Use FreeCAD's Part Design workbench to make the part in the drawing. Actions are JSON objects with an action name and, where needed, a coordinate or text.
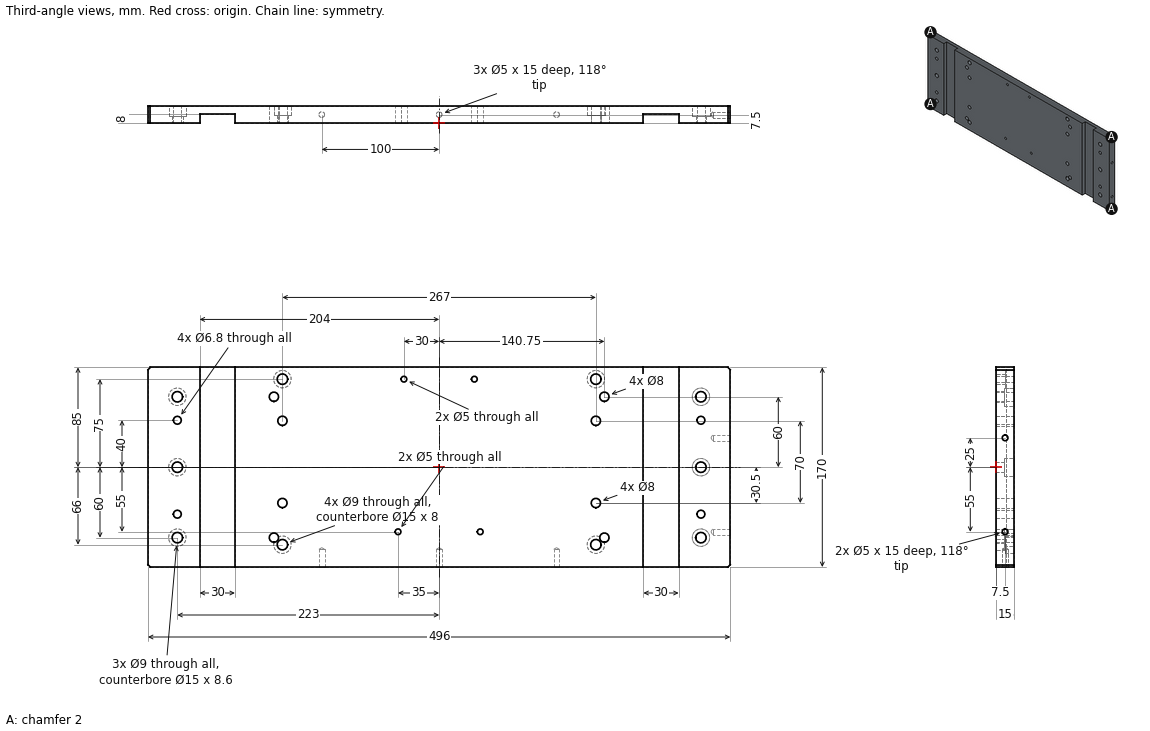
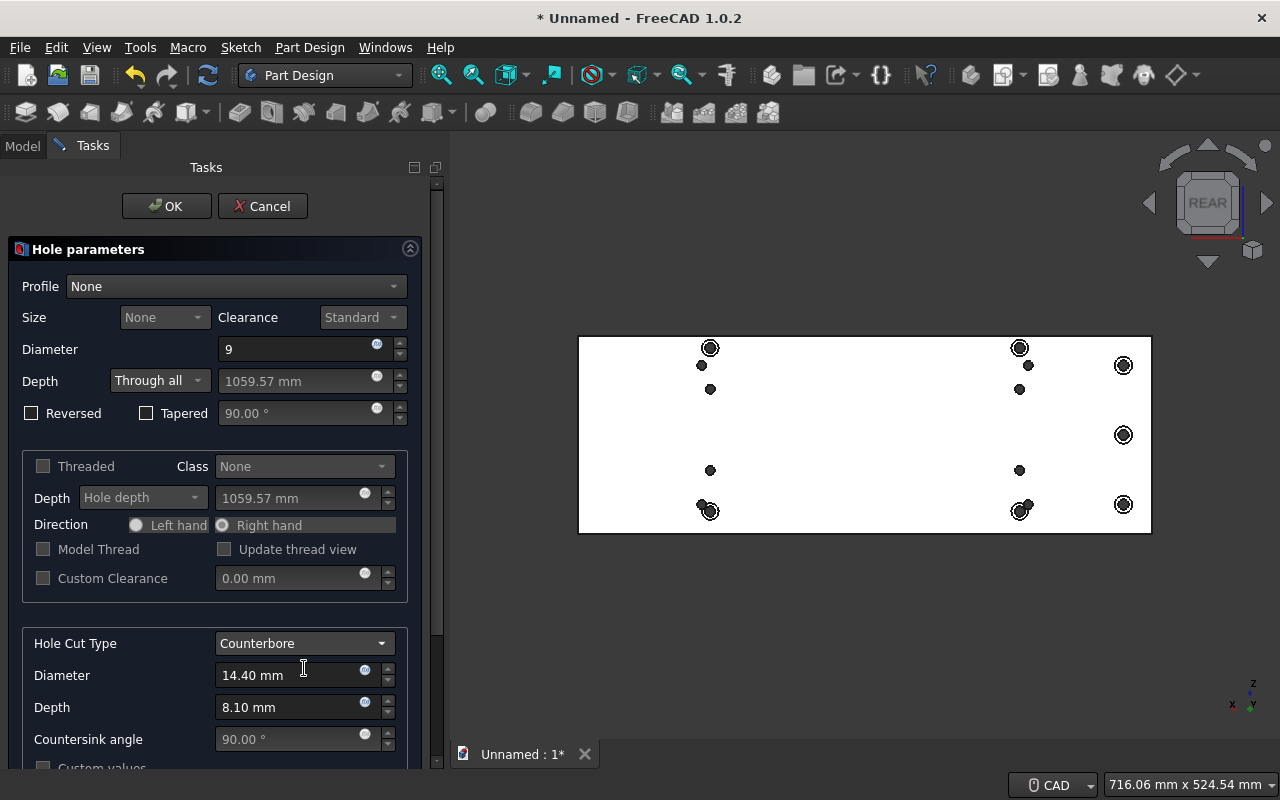
{"action": "triple_click", "coordinate": [298, 675]}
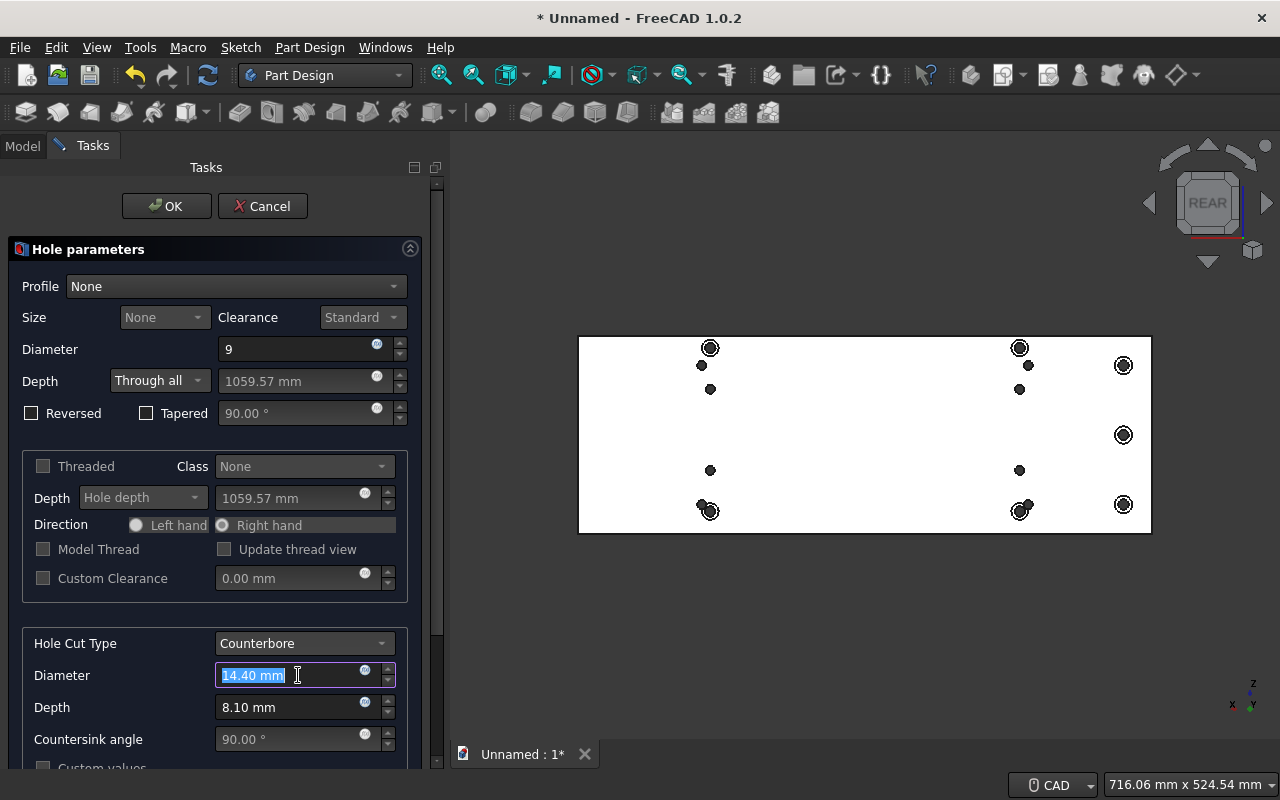
{"action": "type", "text": "15"}
{"action": "key", "text": "Tab"}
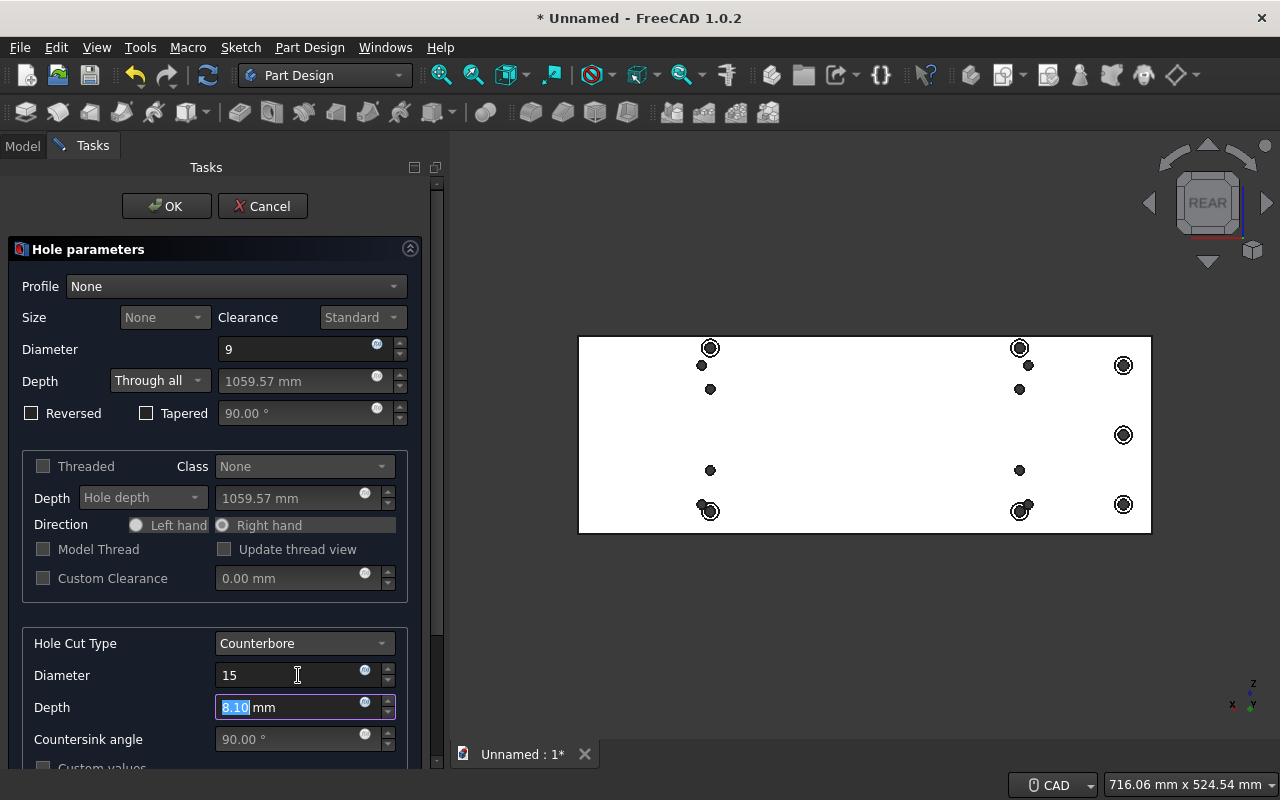
{"action": "type", "text": "8"}
{"action": "key", "text": "Tab"}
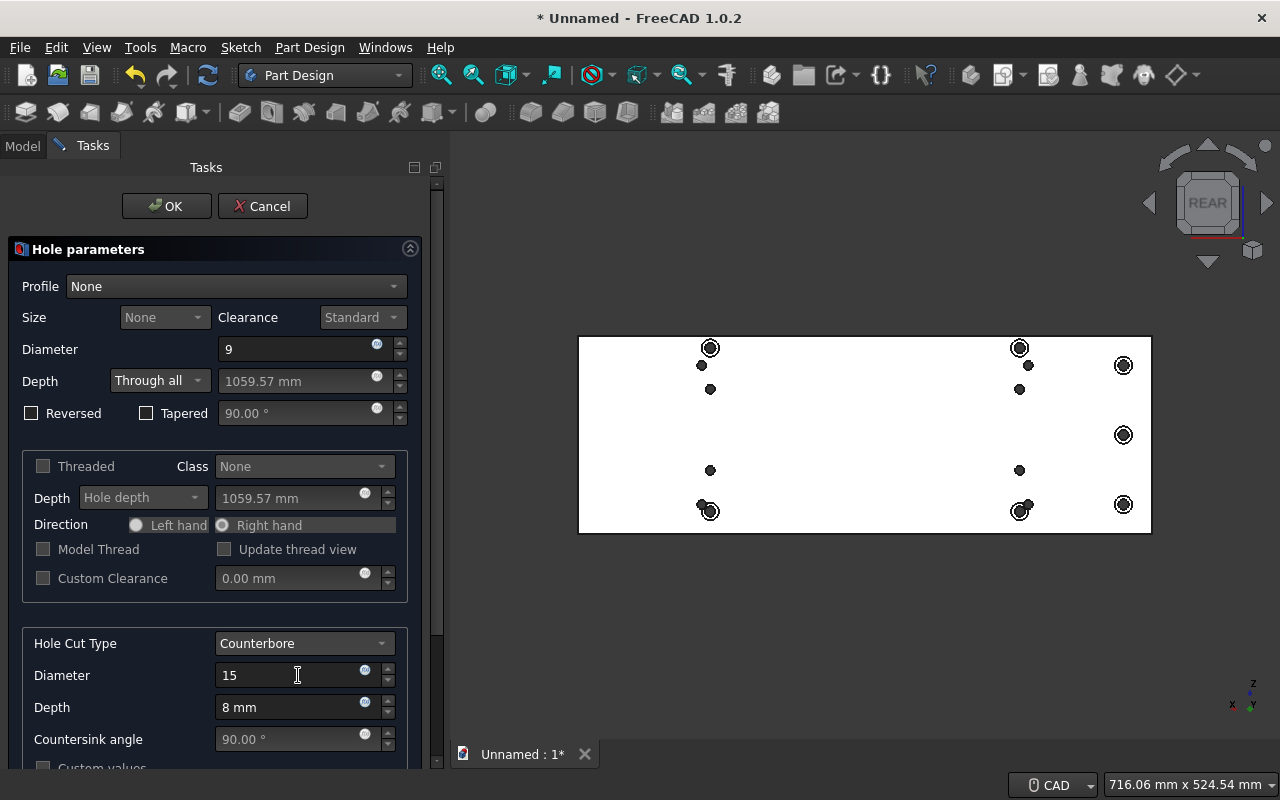
{"action": "left_click", "coordinate": [167, 206]}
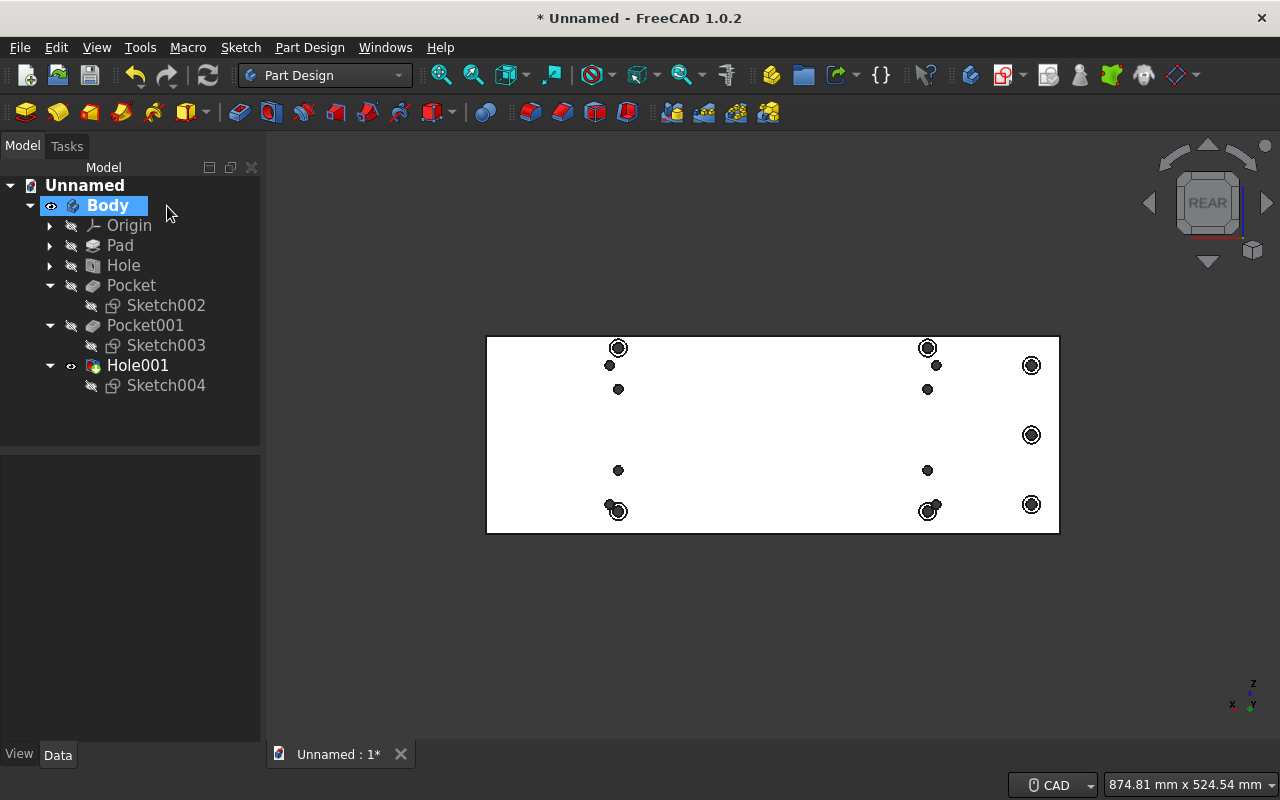
{"action": "key", "text": "0"}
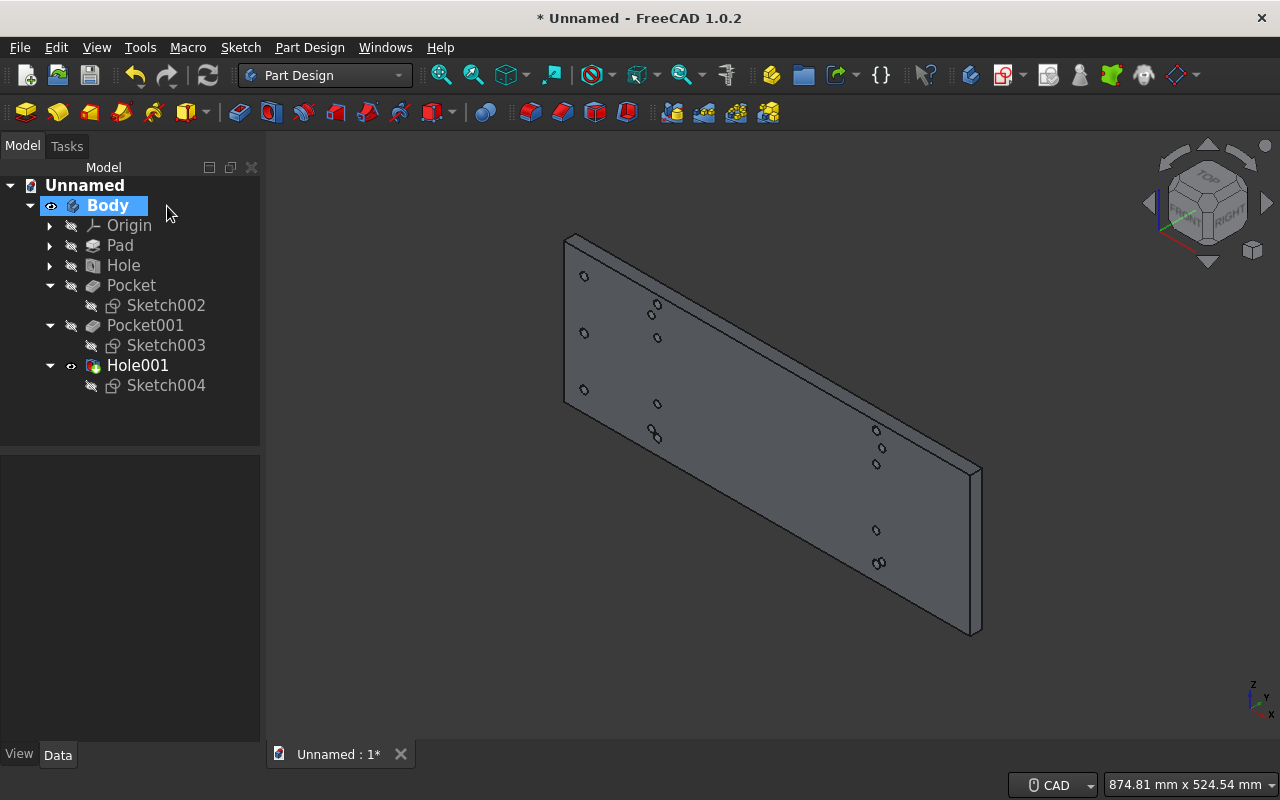
{"action": "key", "text": "3"}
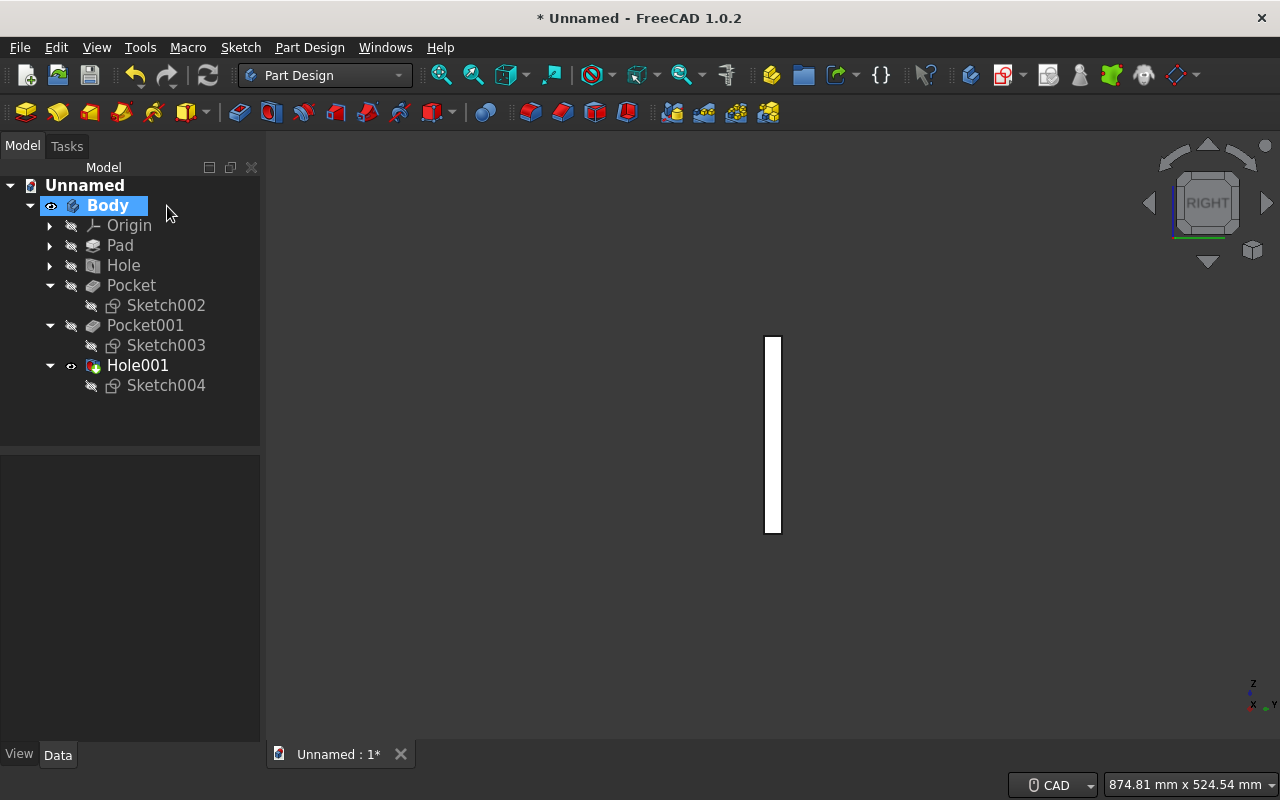
{"action": "left_click", "coordinate": [442, 76]}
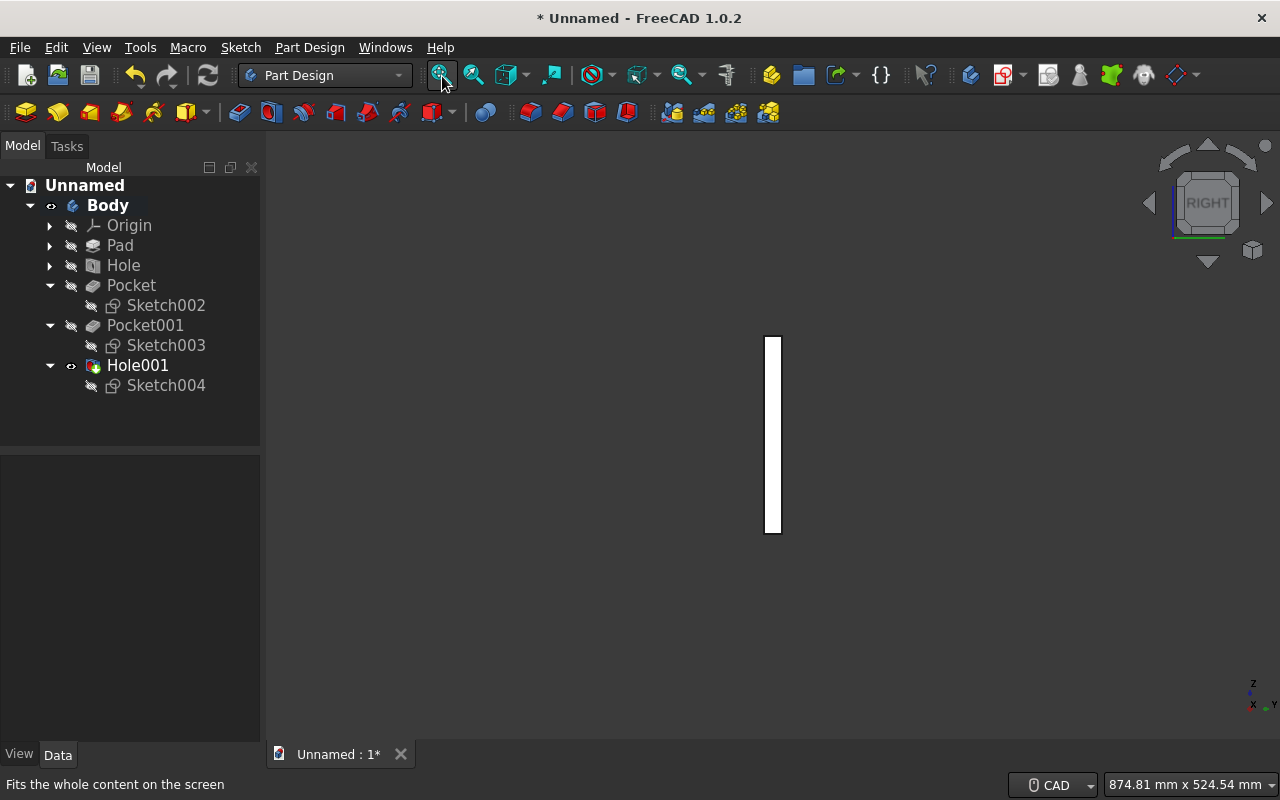
{"action": "left_click", "coordinate": [773, 350]}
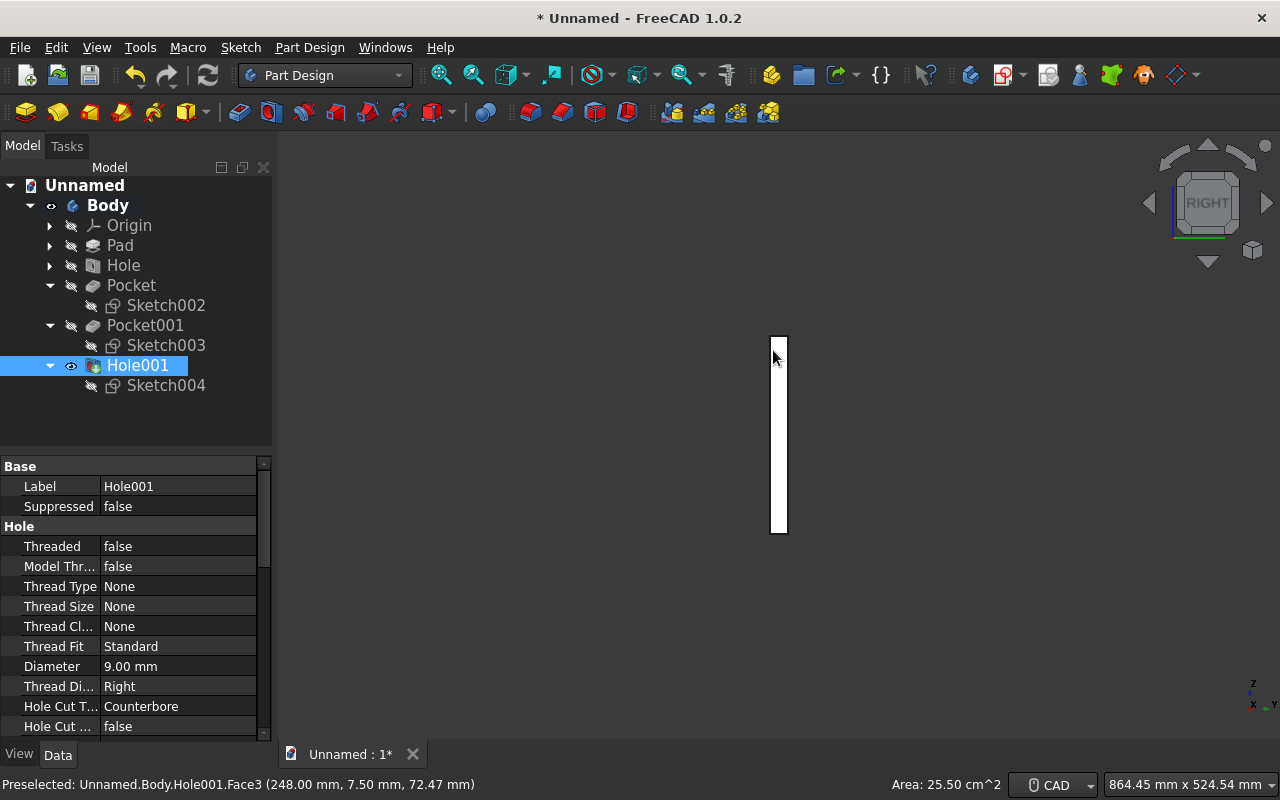
{"action": "left_click", "coordinate": [1004, 76]}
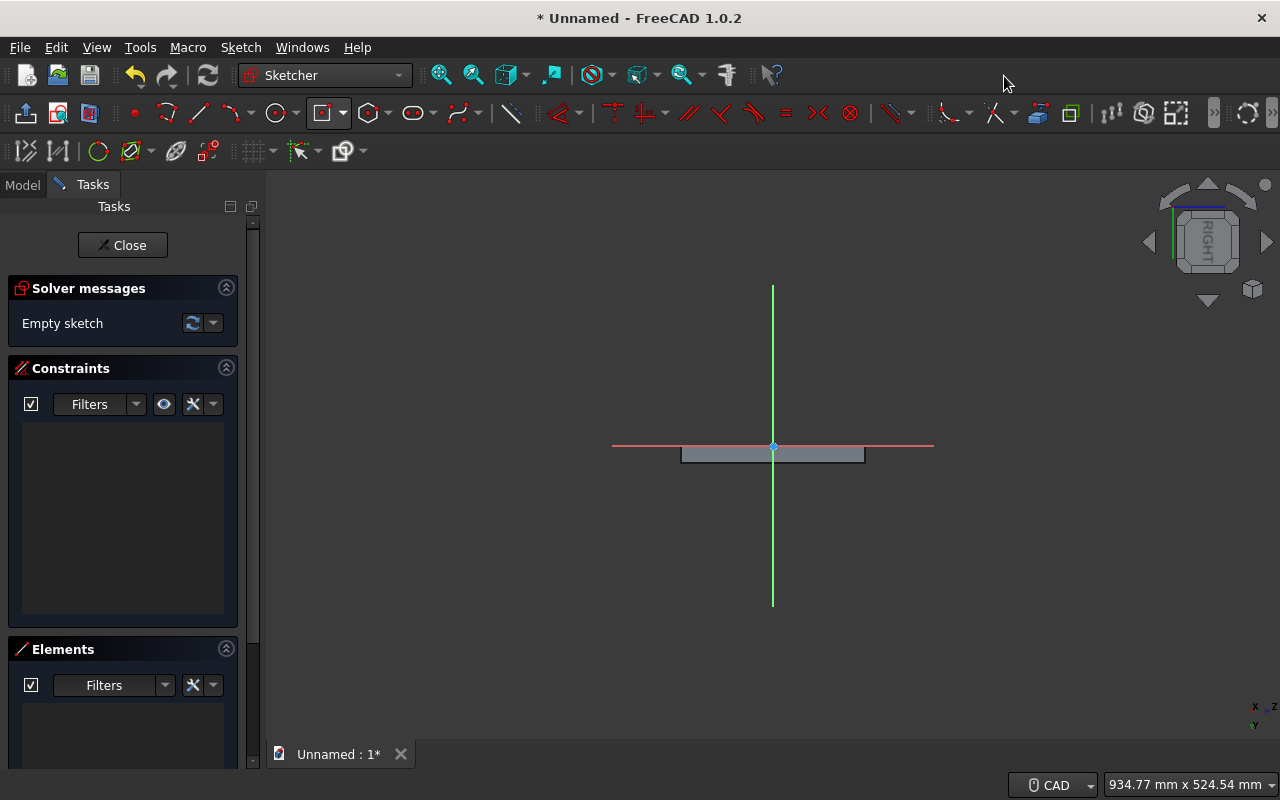
{"action": "scroll", "coordinate": [767, 451], "scroll_direction": "up", "scroll_amount": 9}